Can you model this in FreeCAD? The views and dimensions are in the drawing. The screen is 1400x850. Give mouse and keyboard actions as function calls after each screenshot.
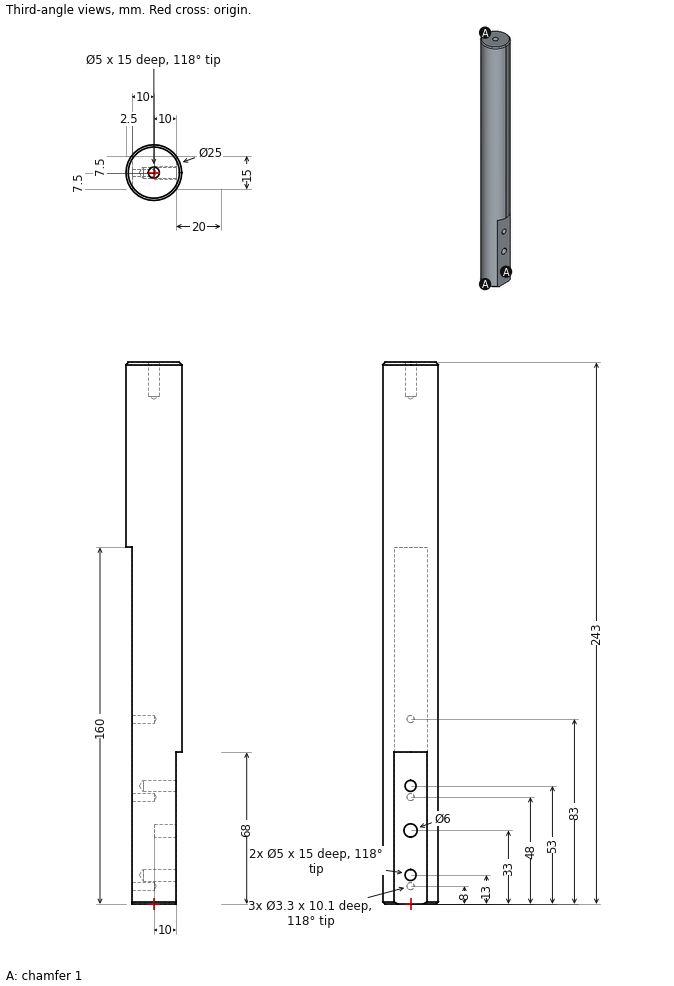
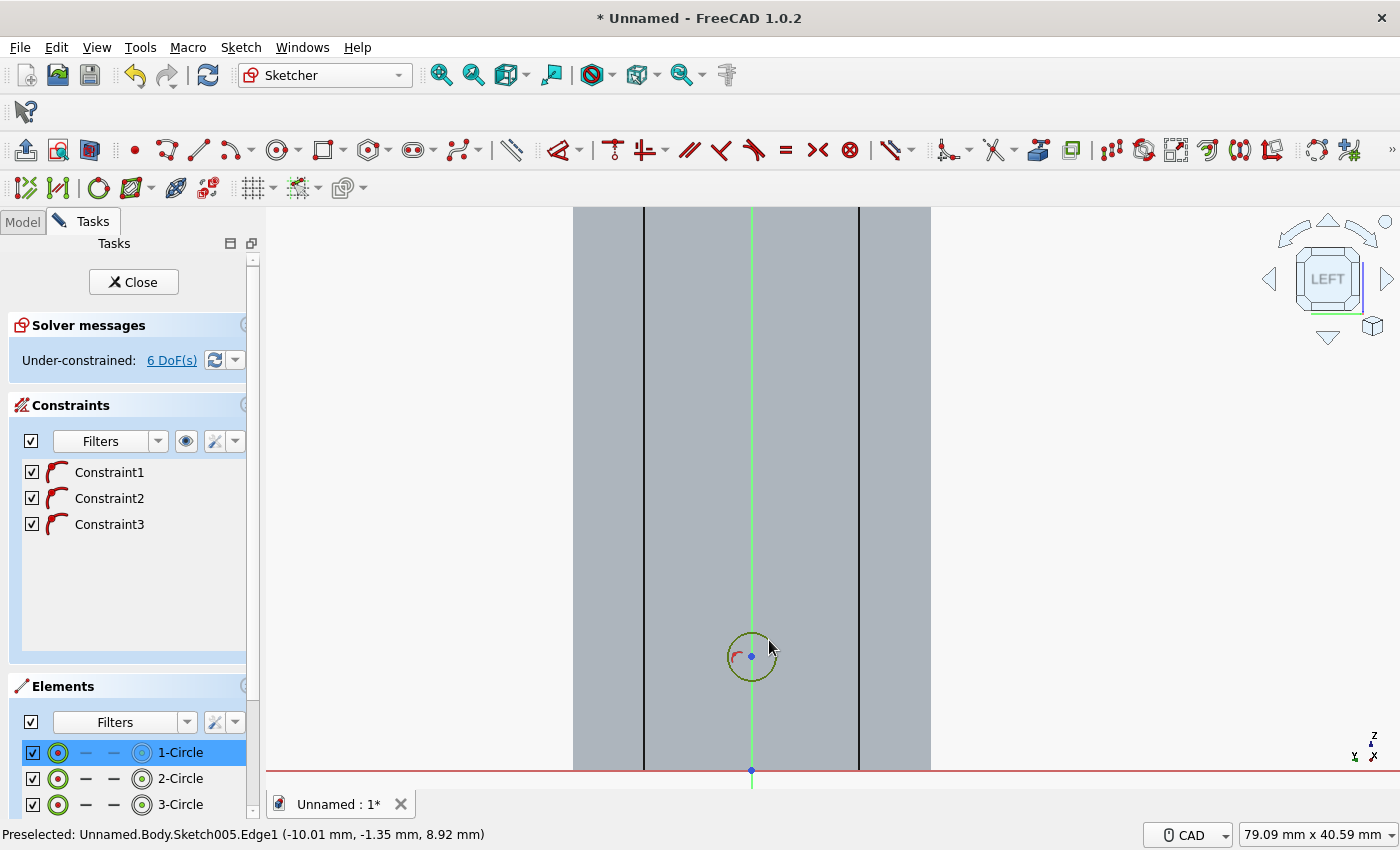
scroll(770, 642, down, 6)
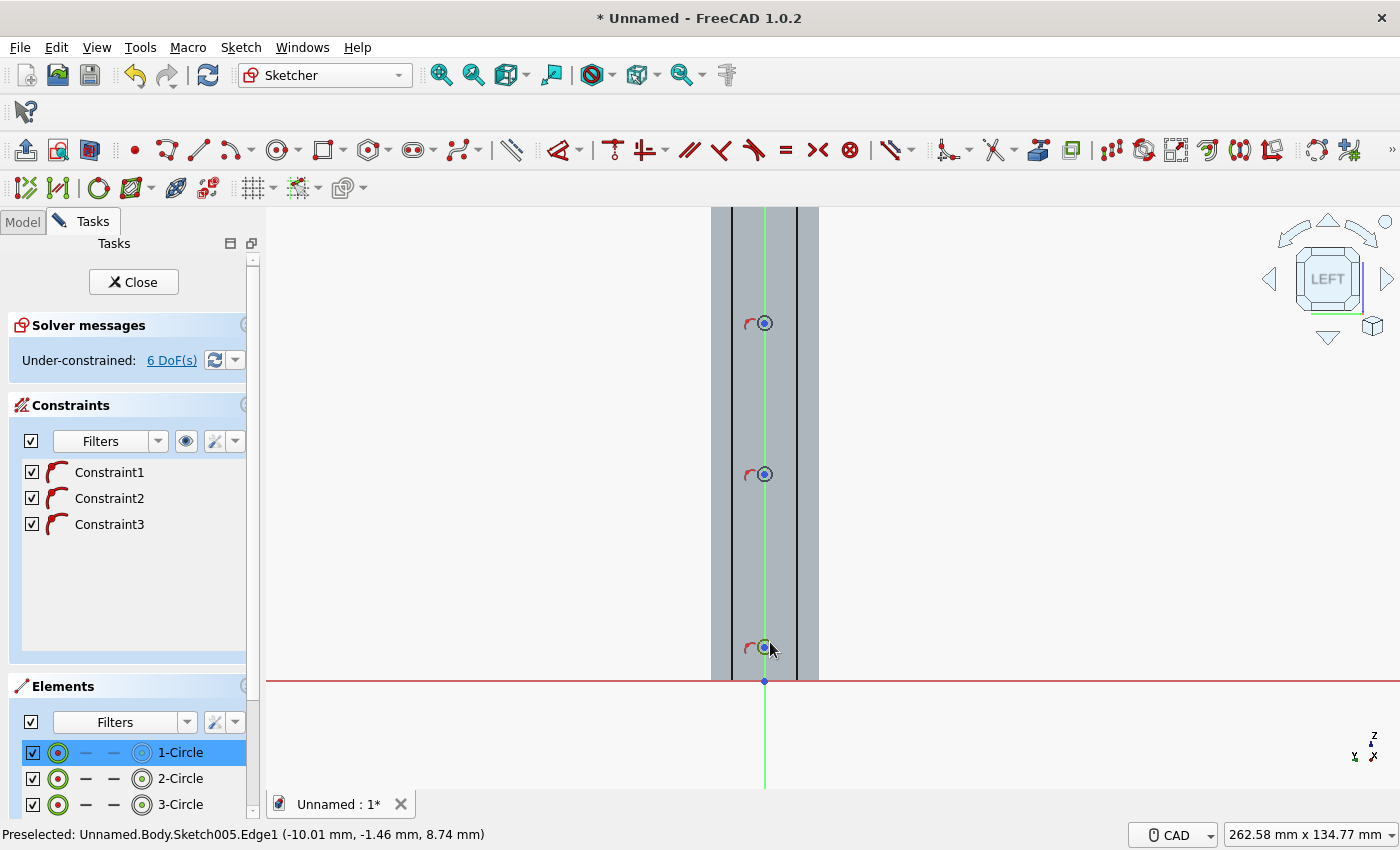
scroll(770, 318, up, 6)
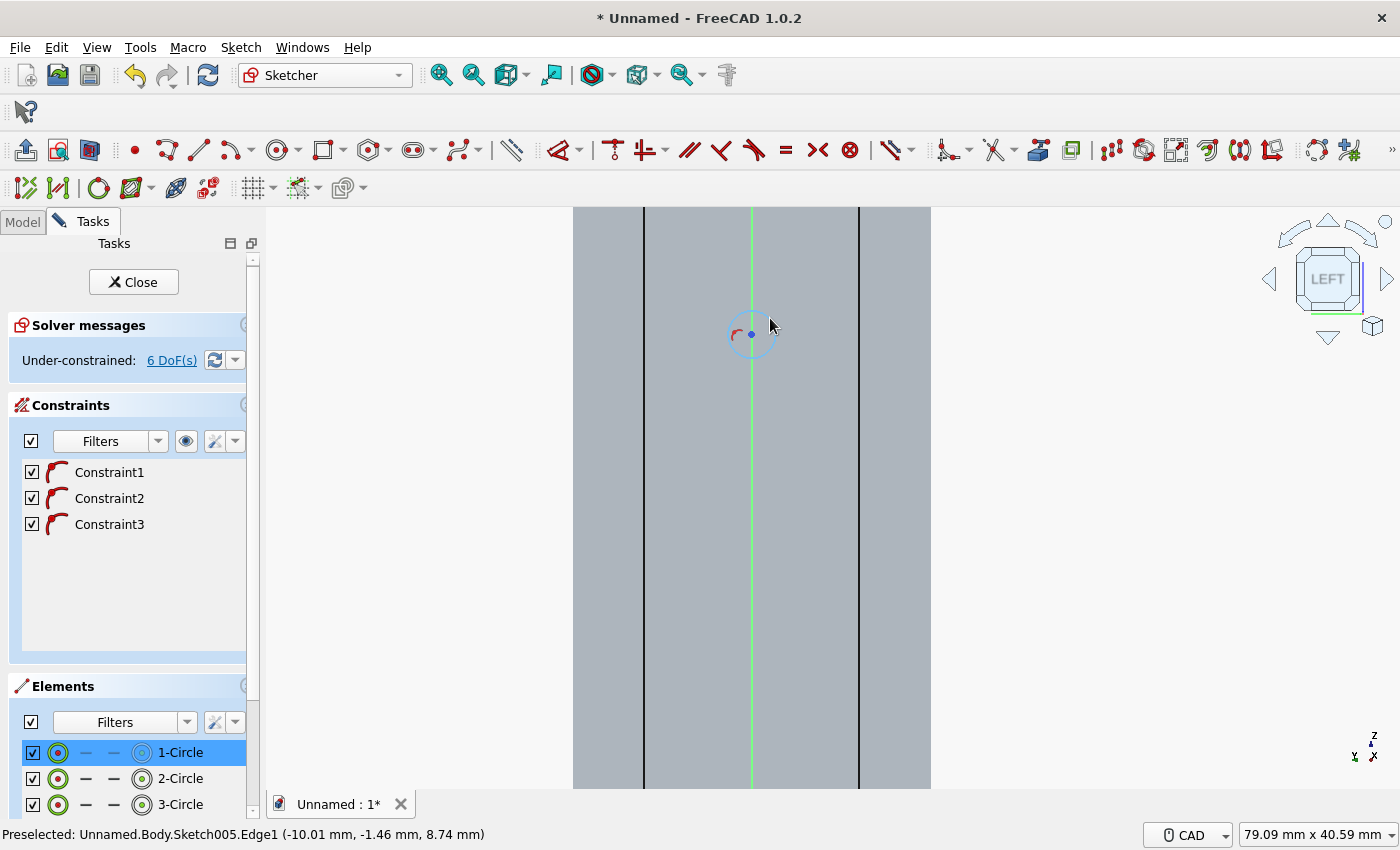
click(769, 318)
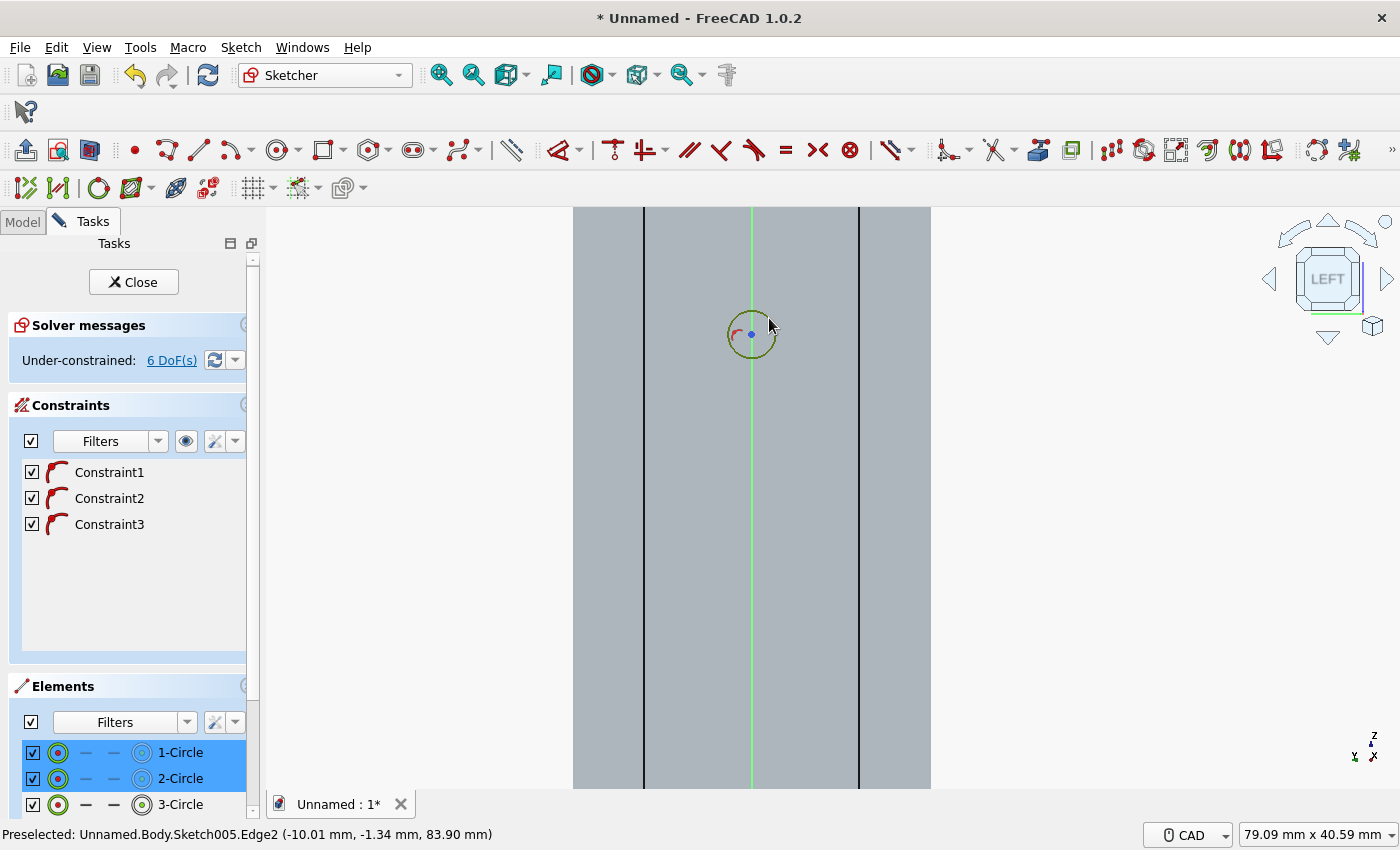
scroll(770, 317, down, 6)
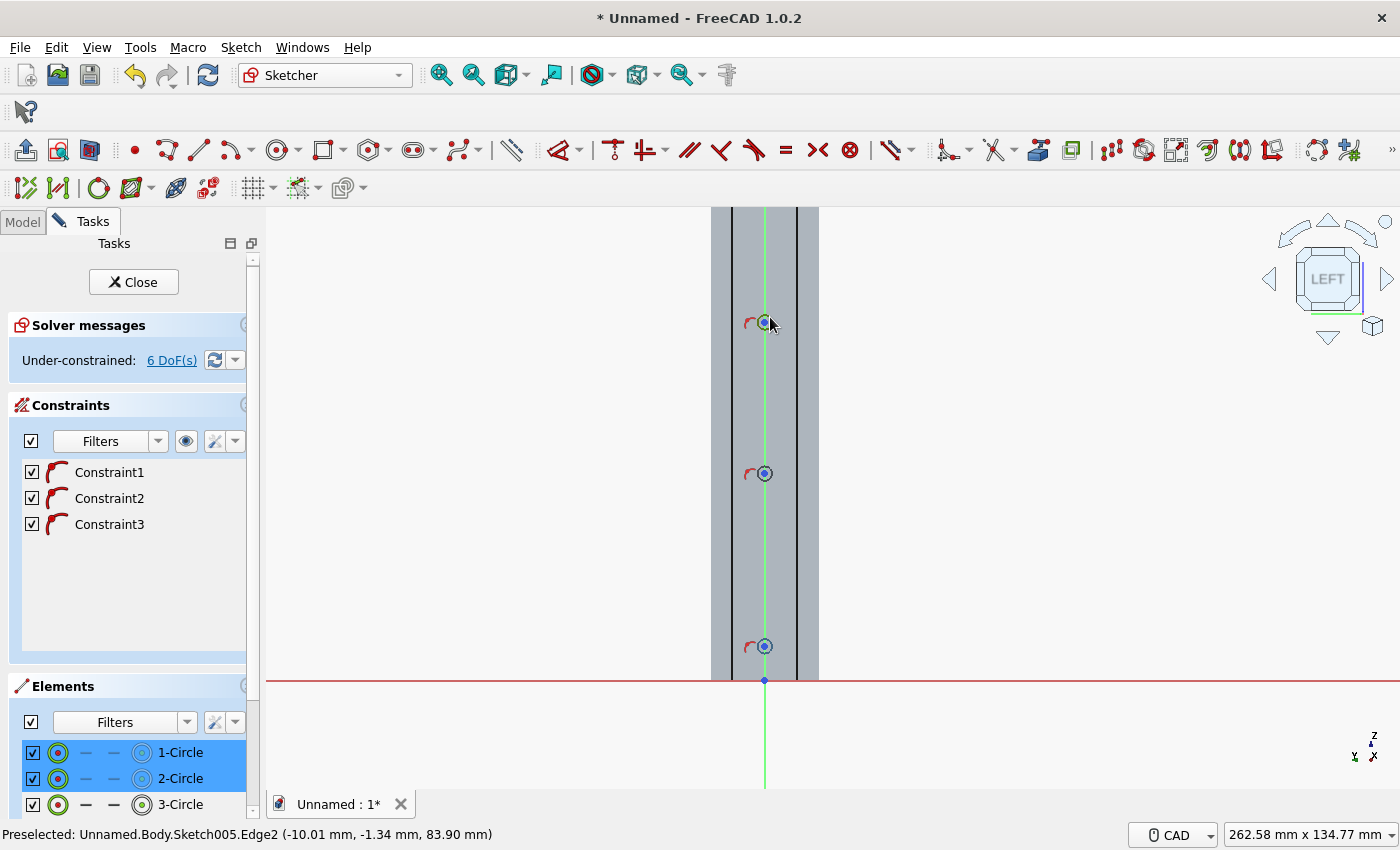
scroll(770, 469, up, 6)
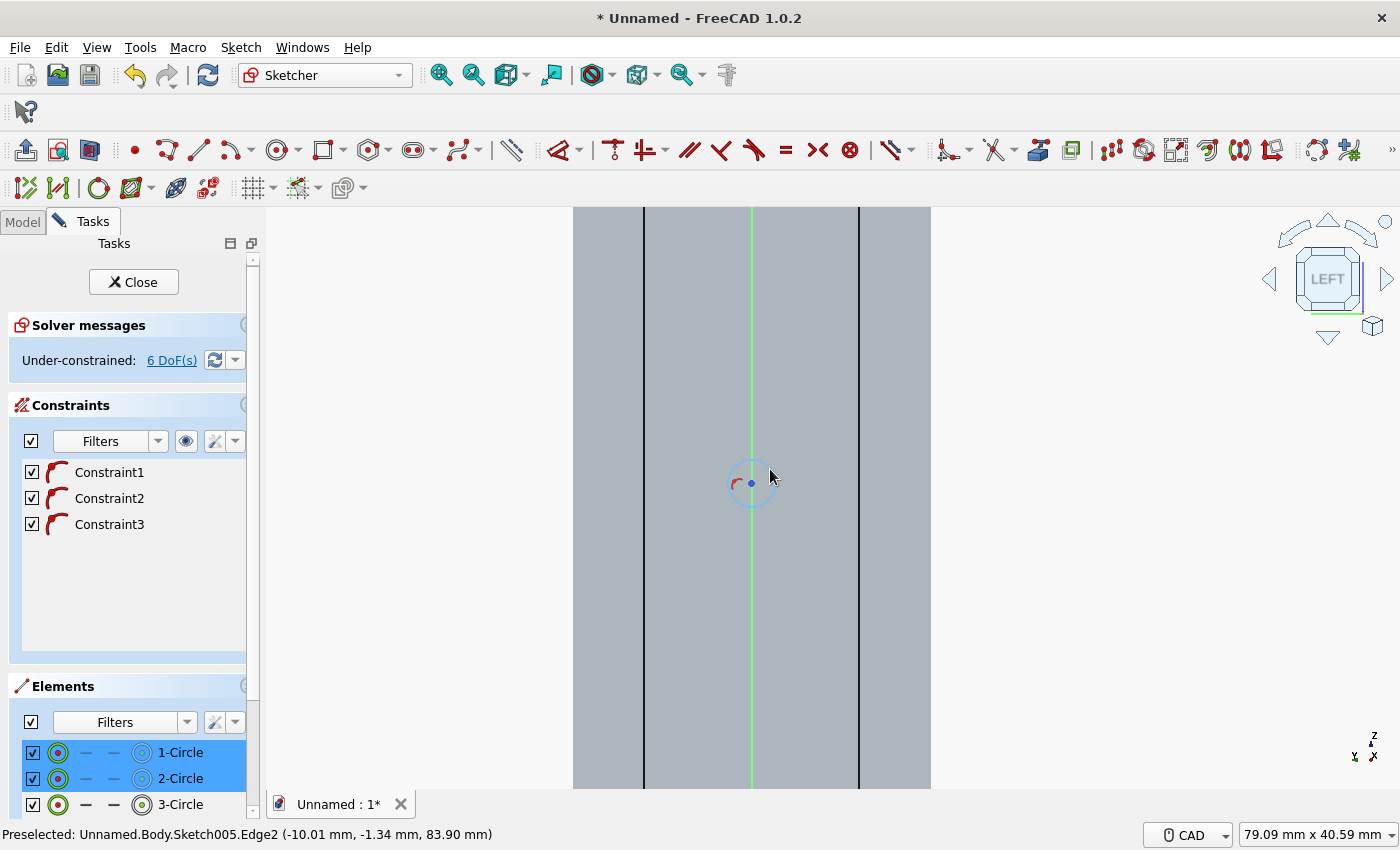
click(769, 466)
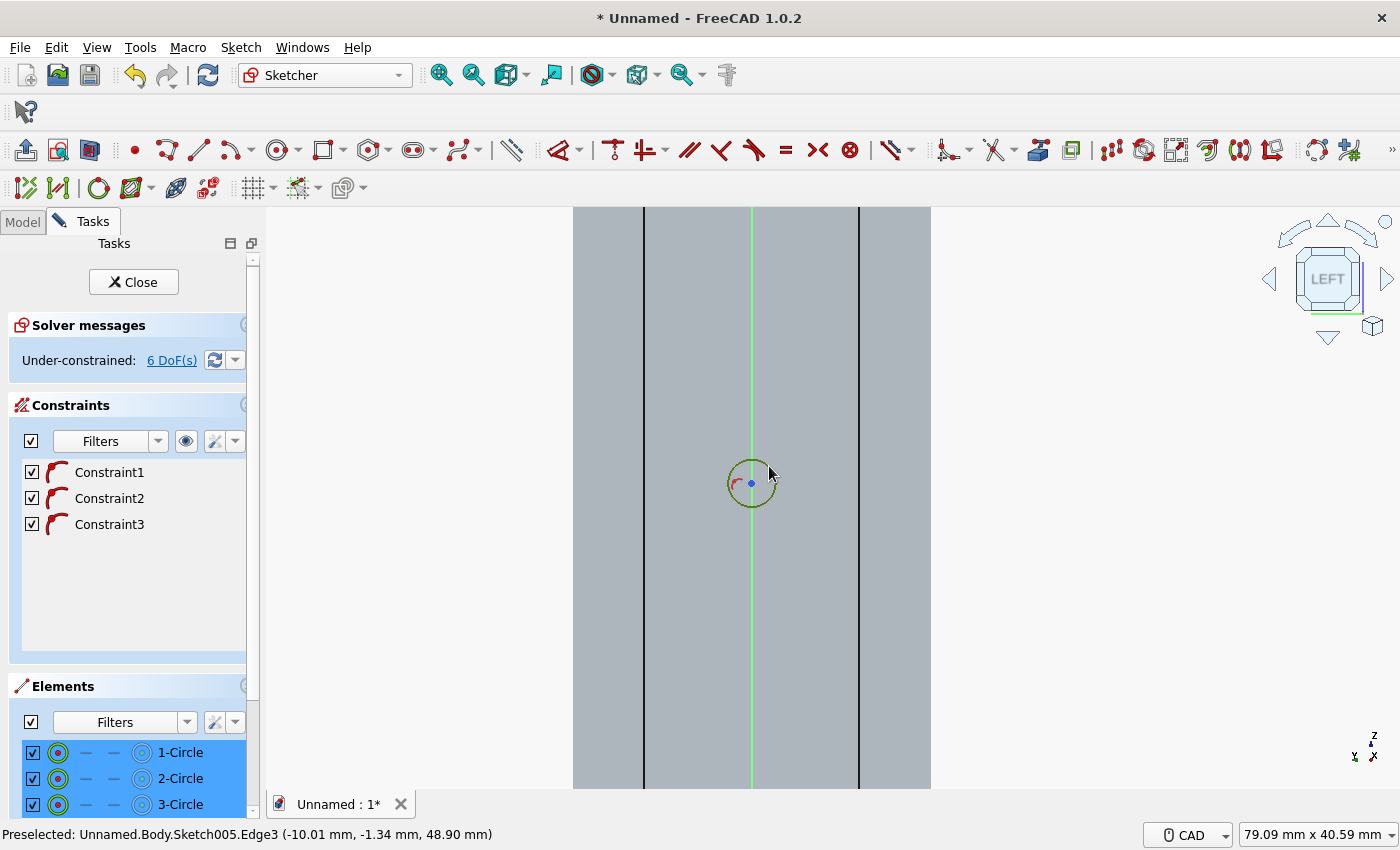
click(786, 150)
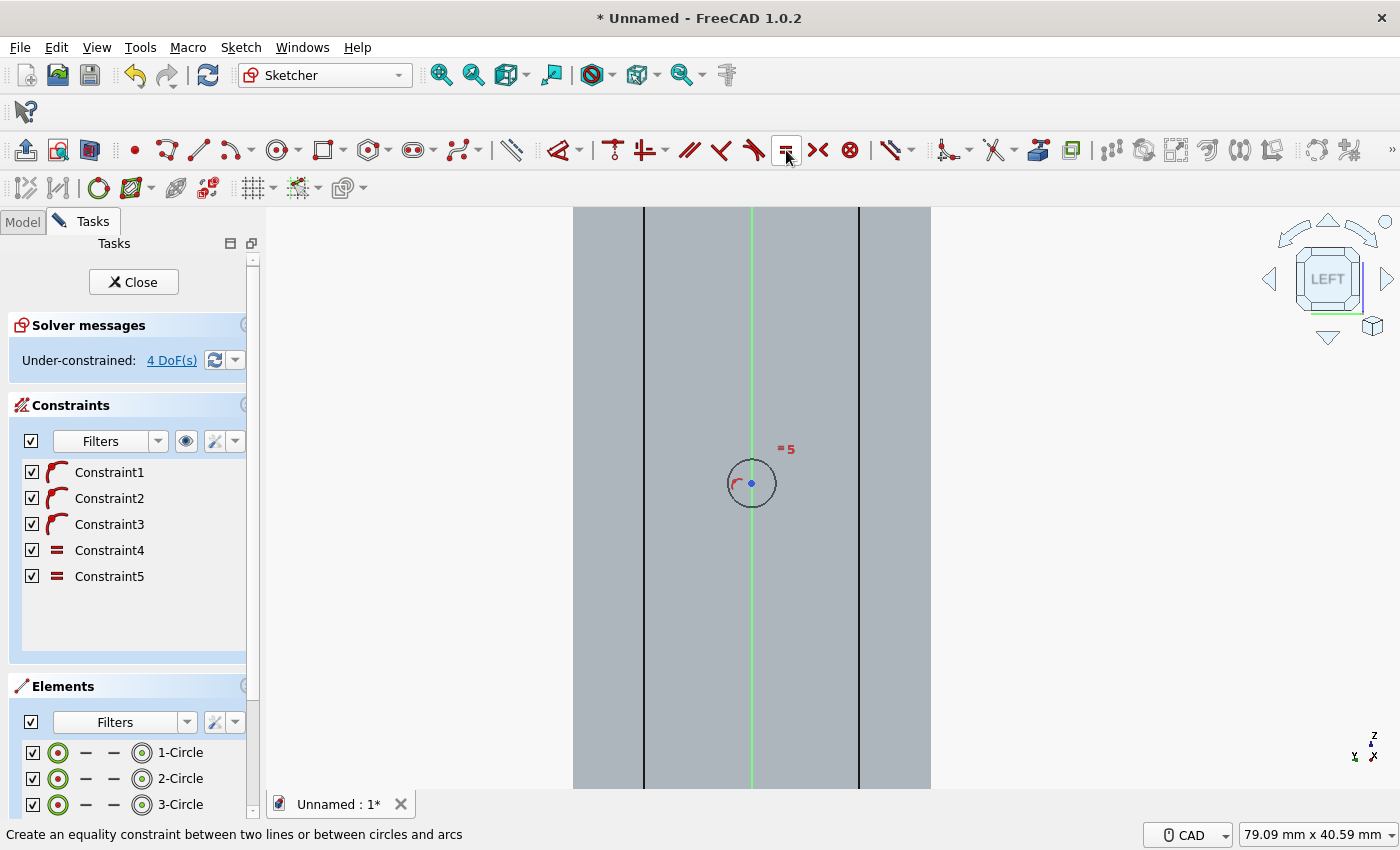
click(558, 150)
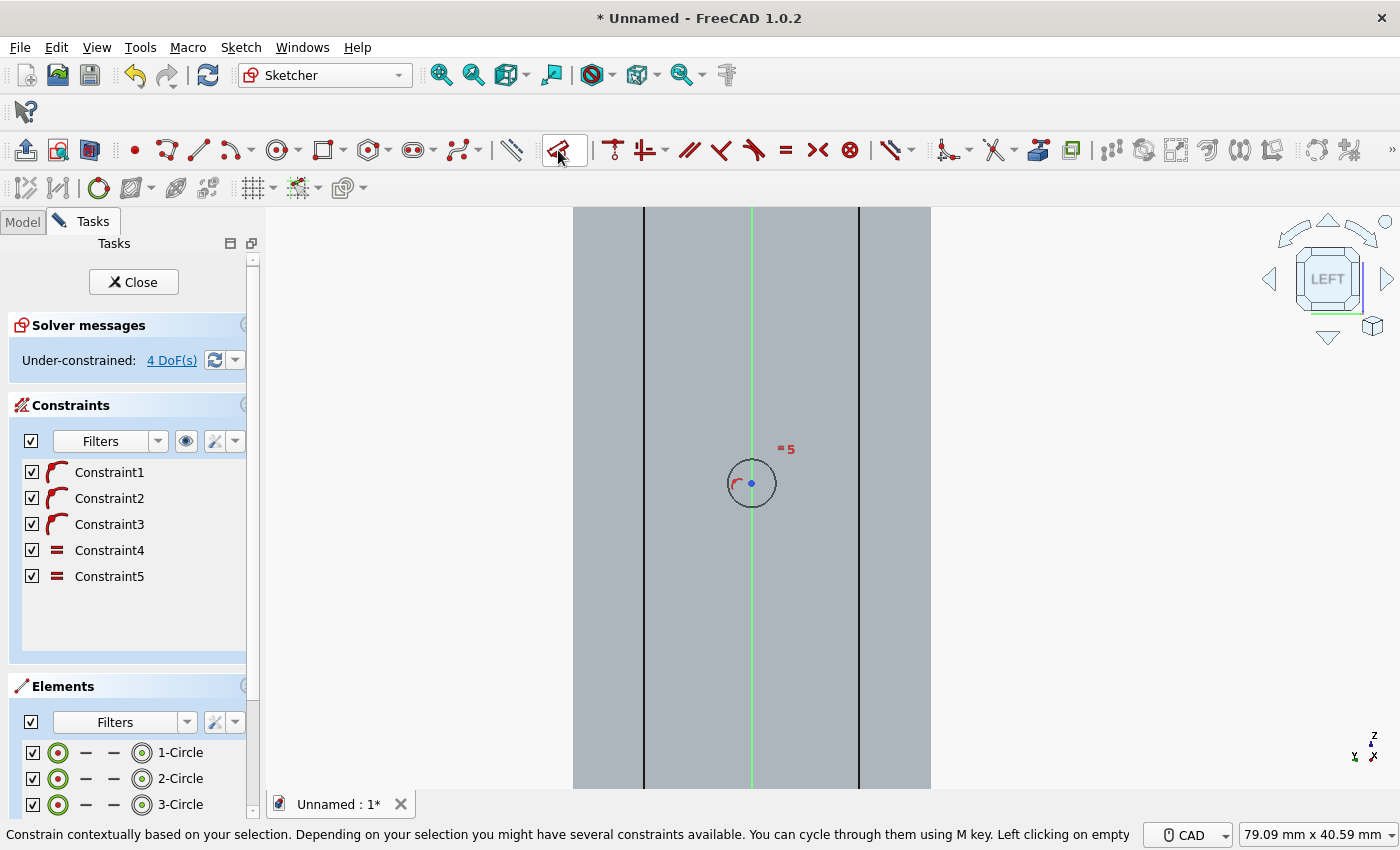
scroll(770, 470, down, 6)